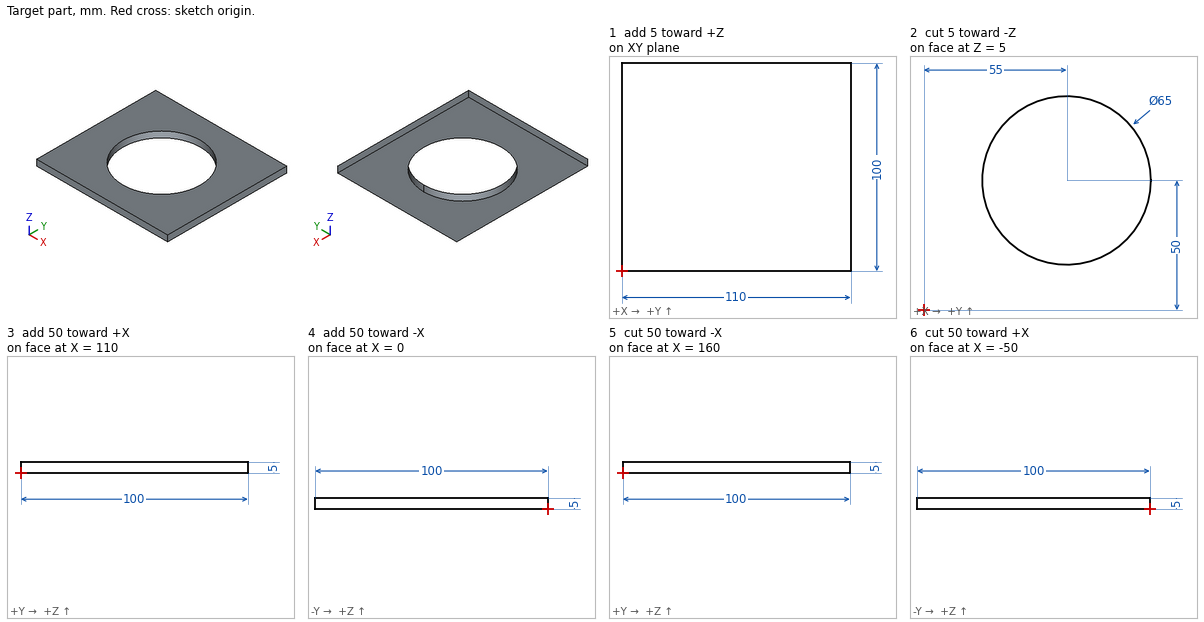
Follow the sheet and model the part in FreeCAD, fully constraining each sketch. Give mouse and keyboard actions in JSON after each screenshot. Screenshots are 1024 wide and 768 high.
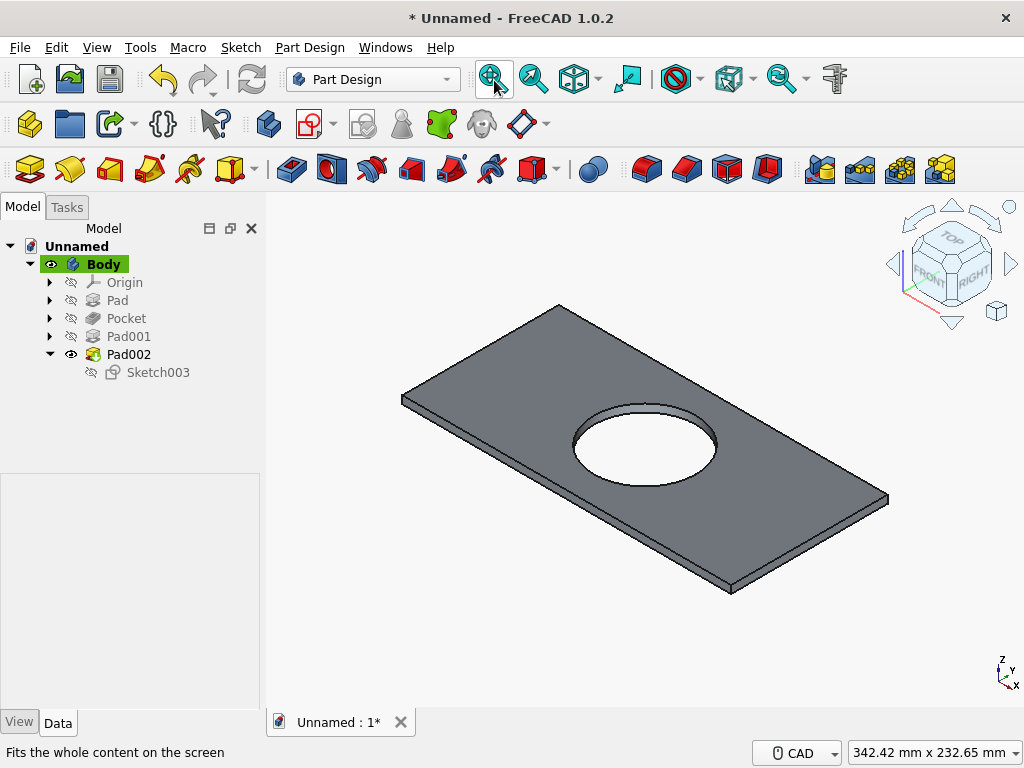
{"action": "key", "text": "3"}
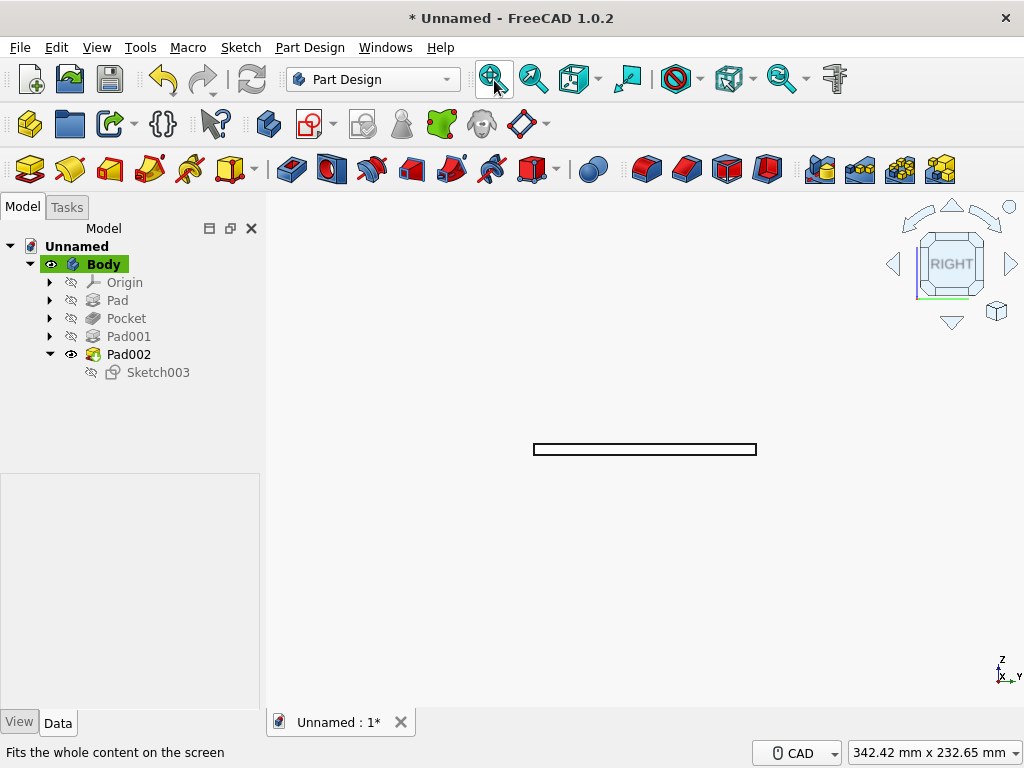
{"action": "left_click", "coordinate": [494, 80]}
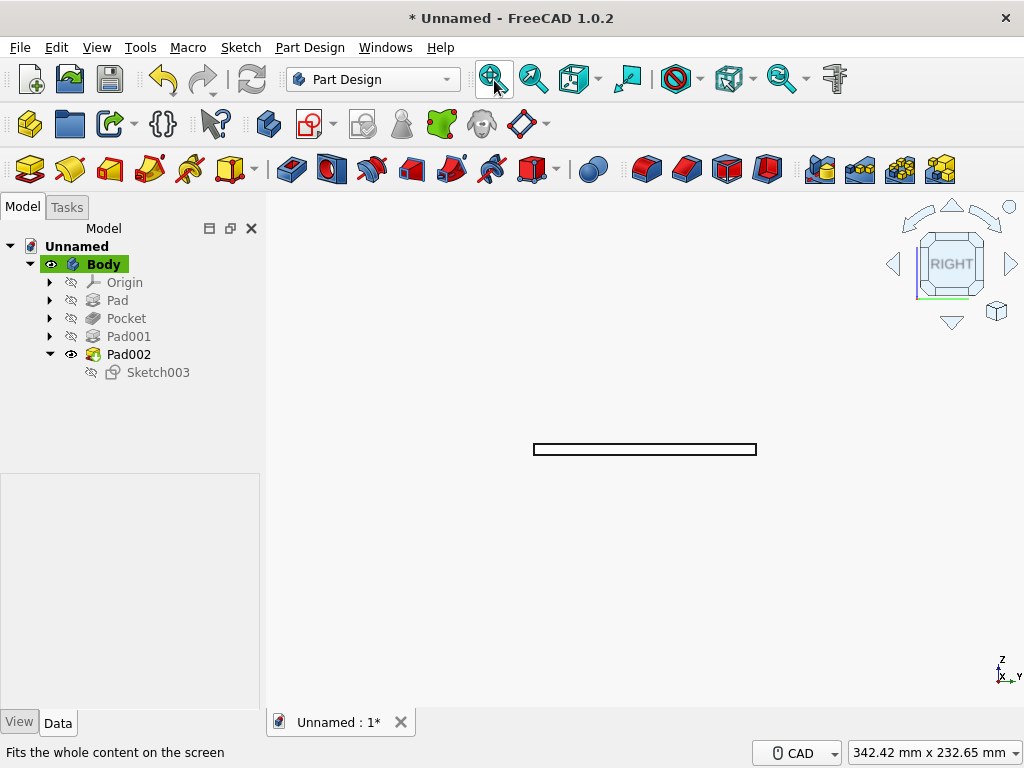
{"action": "scroll", "coordinate": [740, 448], "scroll_direction": "up", "scroll_amount": 4}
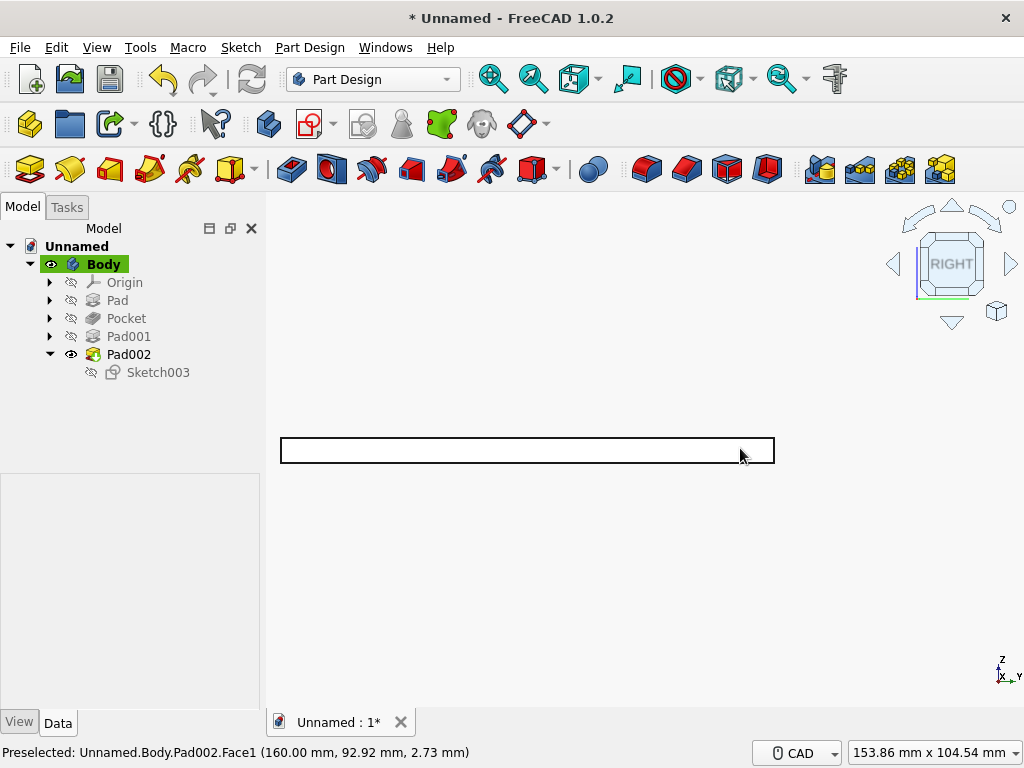
{"action": "left_click", "coordinate": [739, 450]}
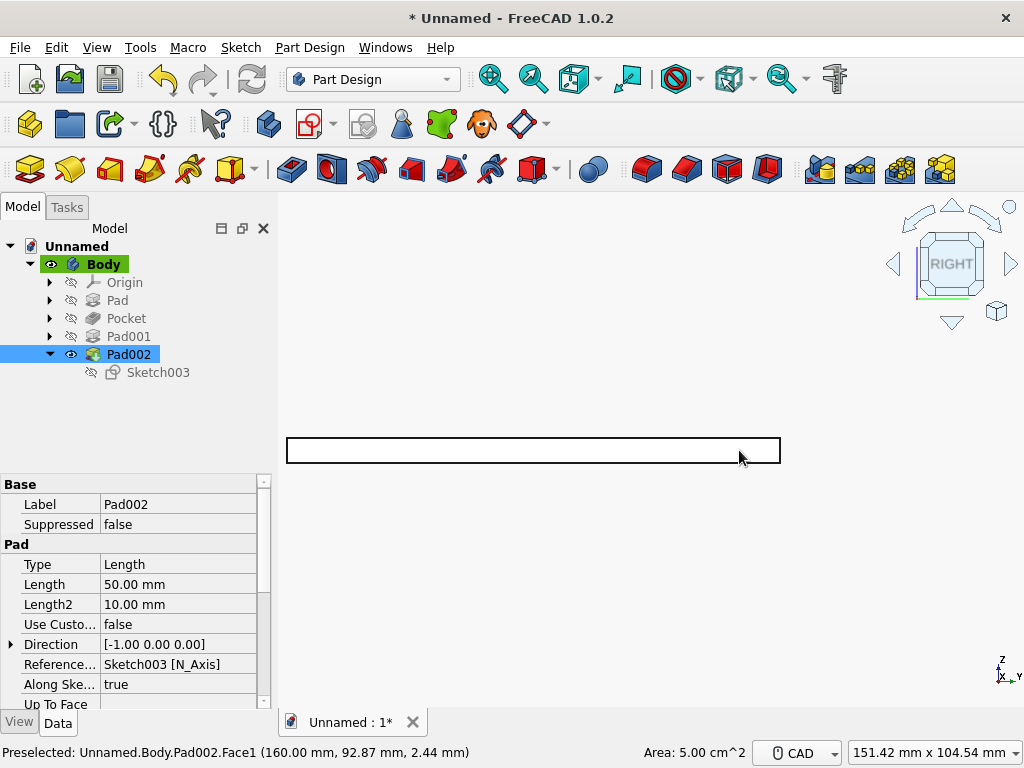
{"action": "left_click", "coordinate": [310, 124]}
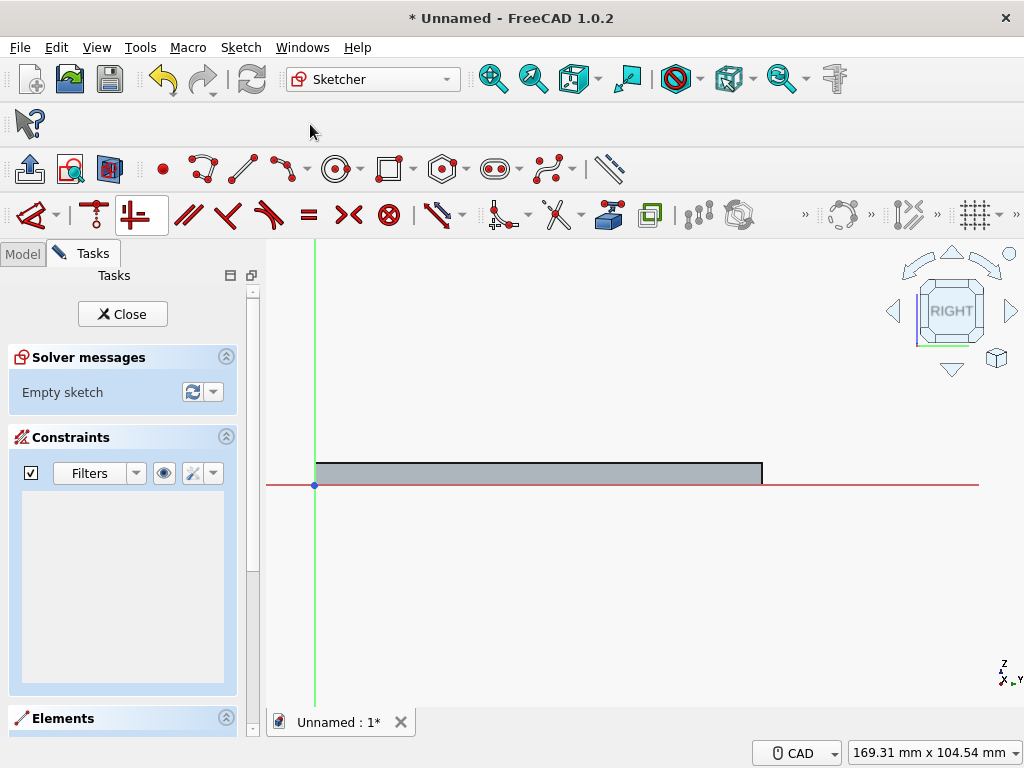
{"action": "scroll", "coordinate": [748, 468], "scroll_direction": "down", "scroll_amount": 1}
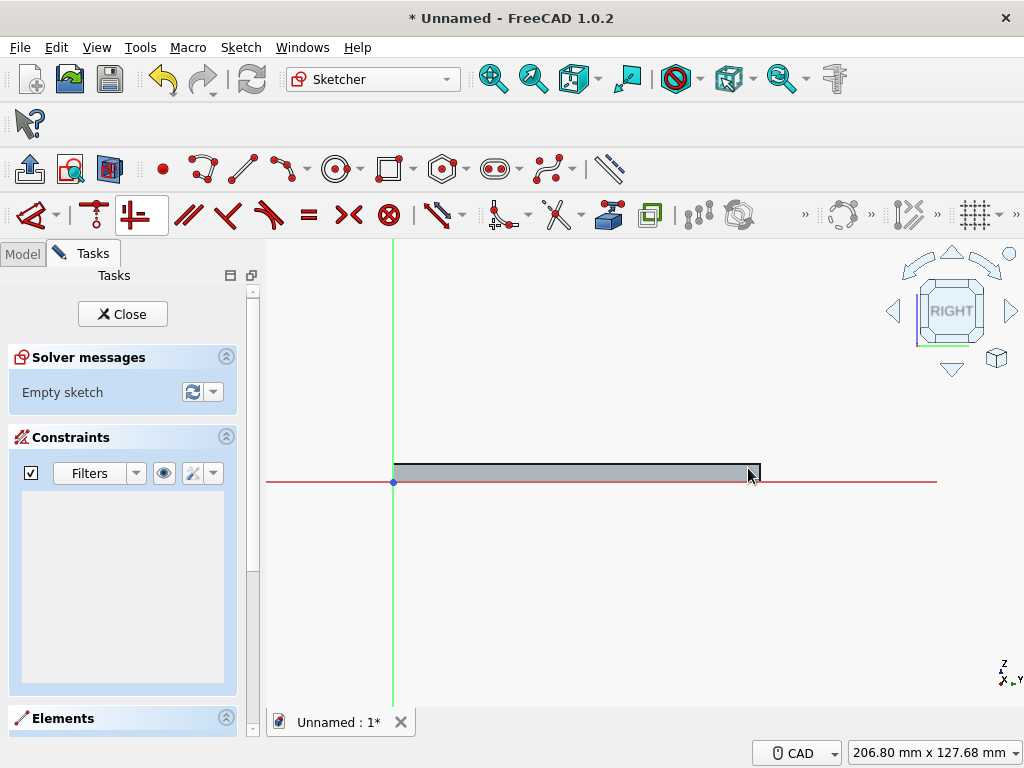
{"action": "left_click", "coordinate": [390, 170]}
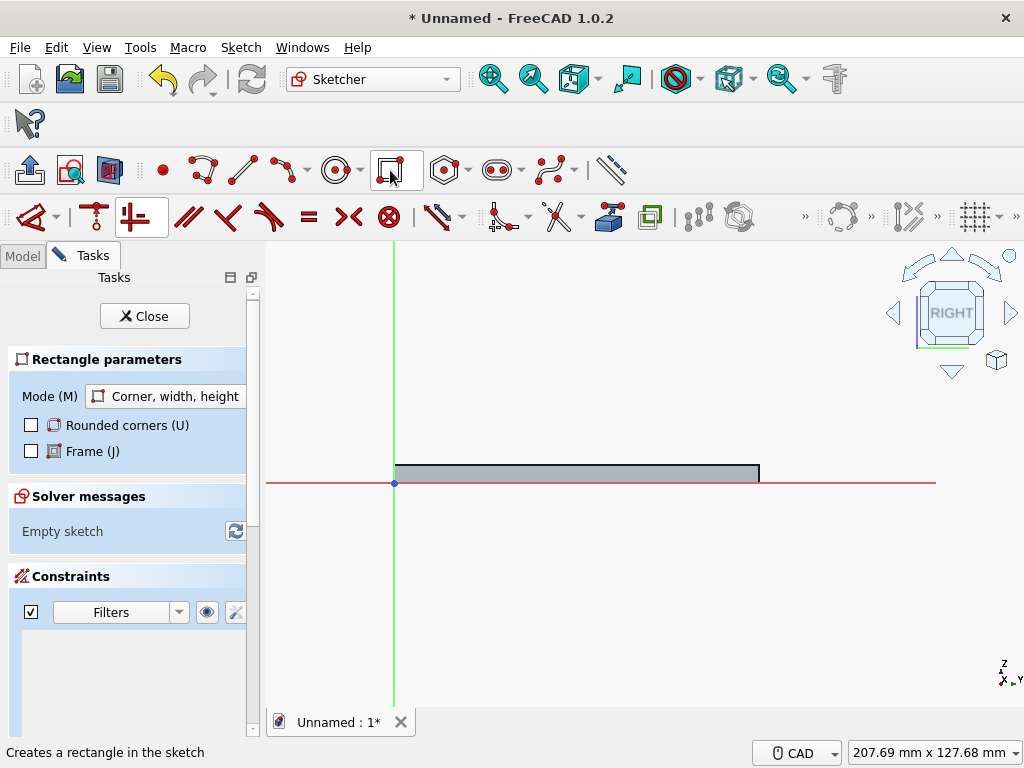
{"action": "left_click", "coordinate": [394, 483]}
{"action": "left_click", "coordinate": [759, 465]}
{"action": "key", "text": "Escape"}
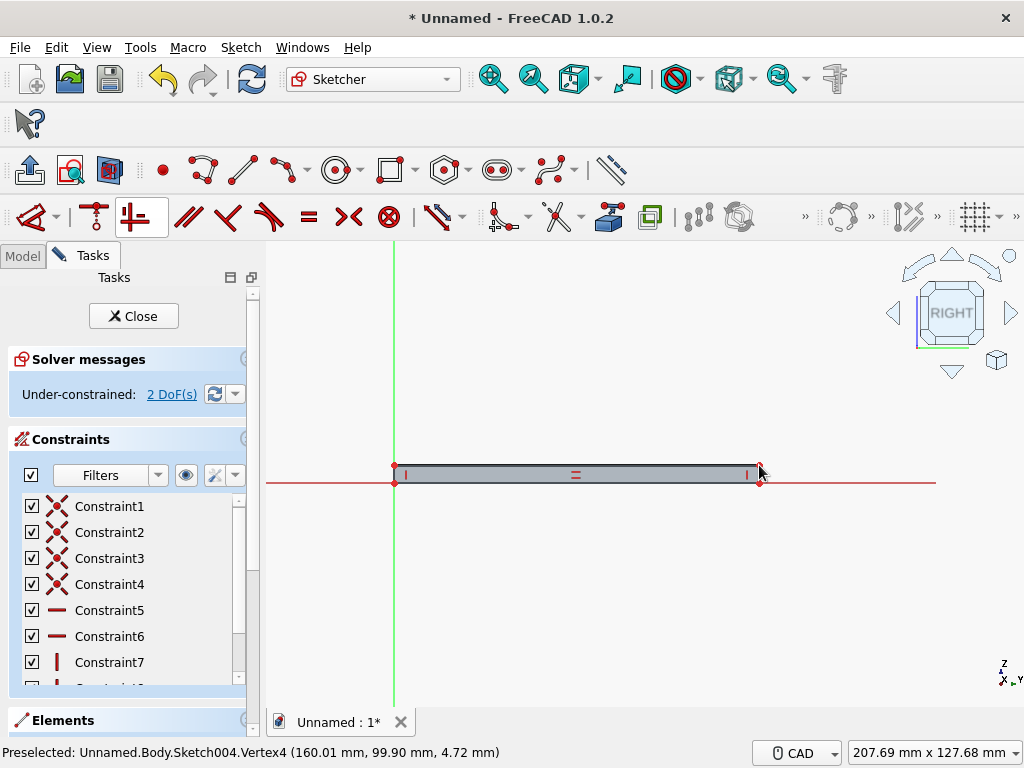
{"action": "left_click", "coordinate": [32, 218]}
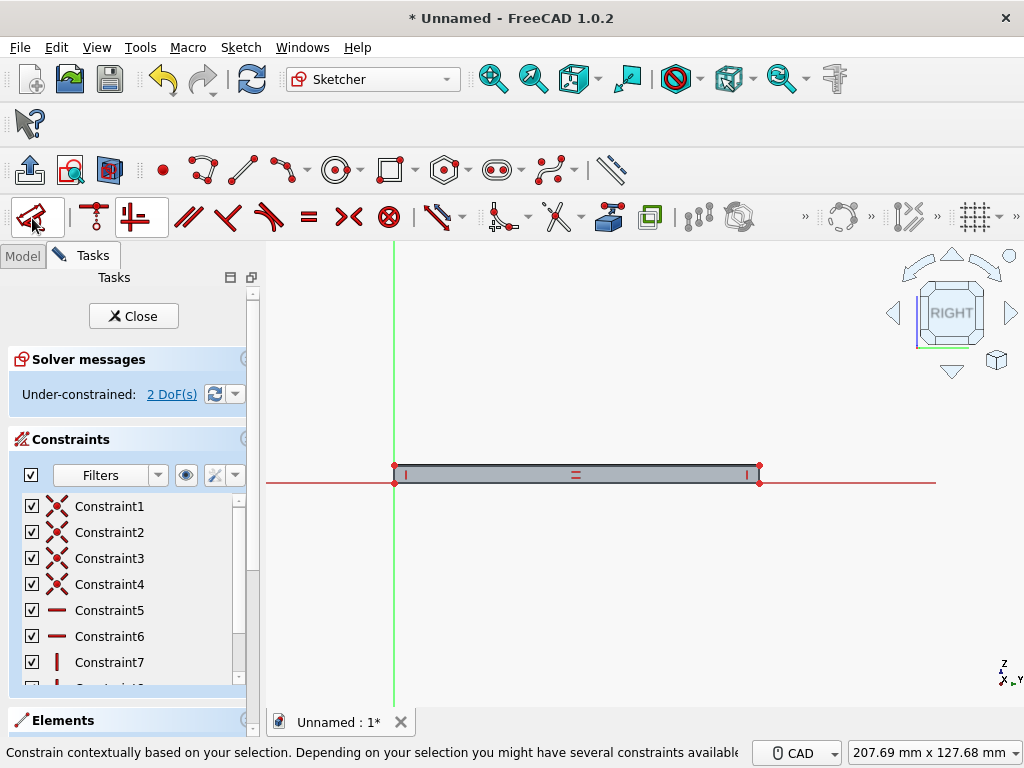
{"action": "scroll", "coordinate": [759, 475], "scroll_direction": "up", "scroll_amount": 4}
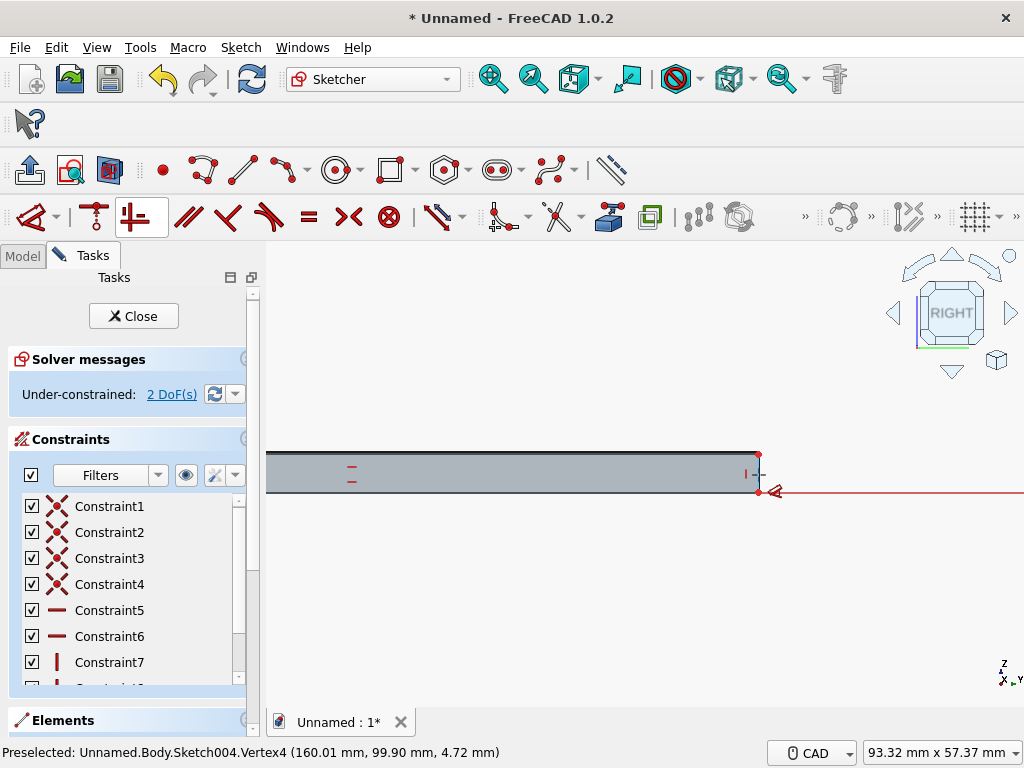
{"action": "left_click", "coordinate": [758, 474]}
{"action": "left_click", "coordinate": [792, 474]}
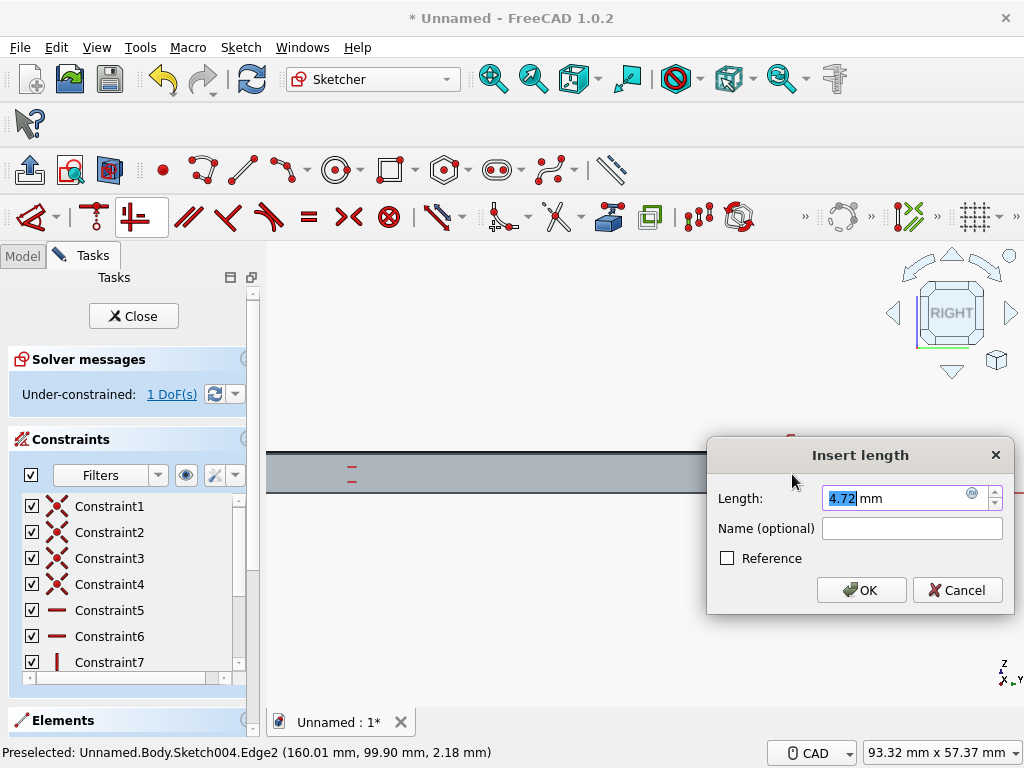
{"action": "type", "text": "5"}
{"action": "key", "text": "Return"}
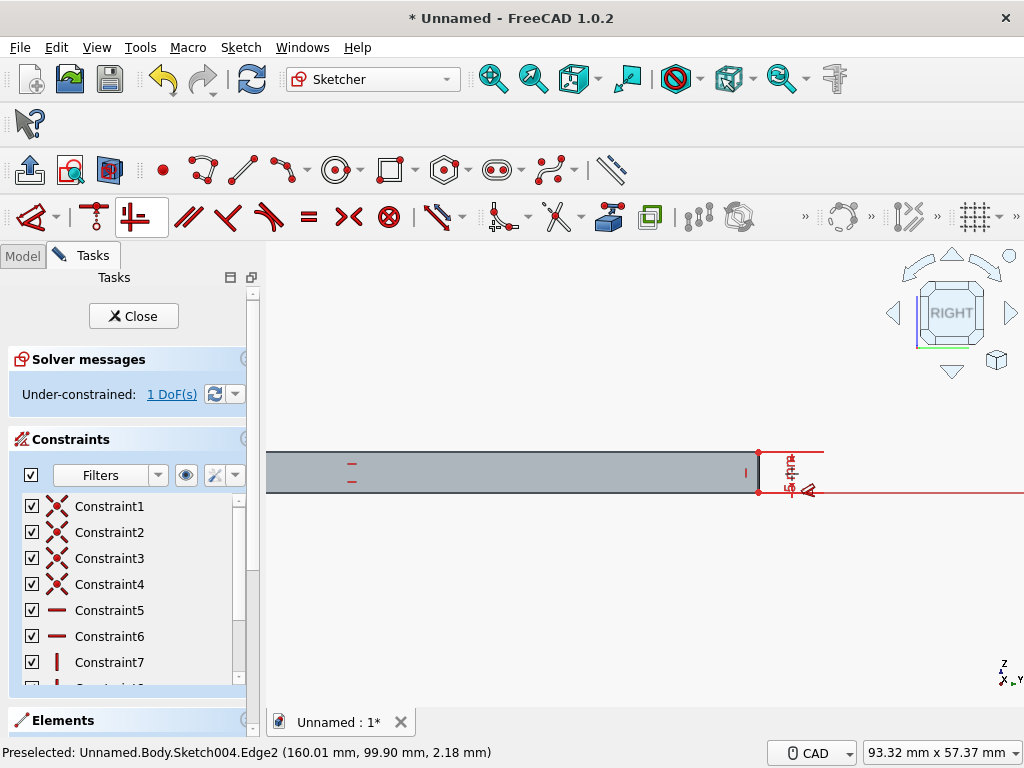
{"action": "left_click", "coordinate": [515, 493]}
{"action": "left_click", "coordinate": [526, 527]}